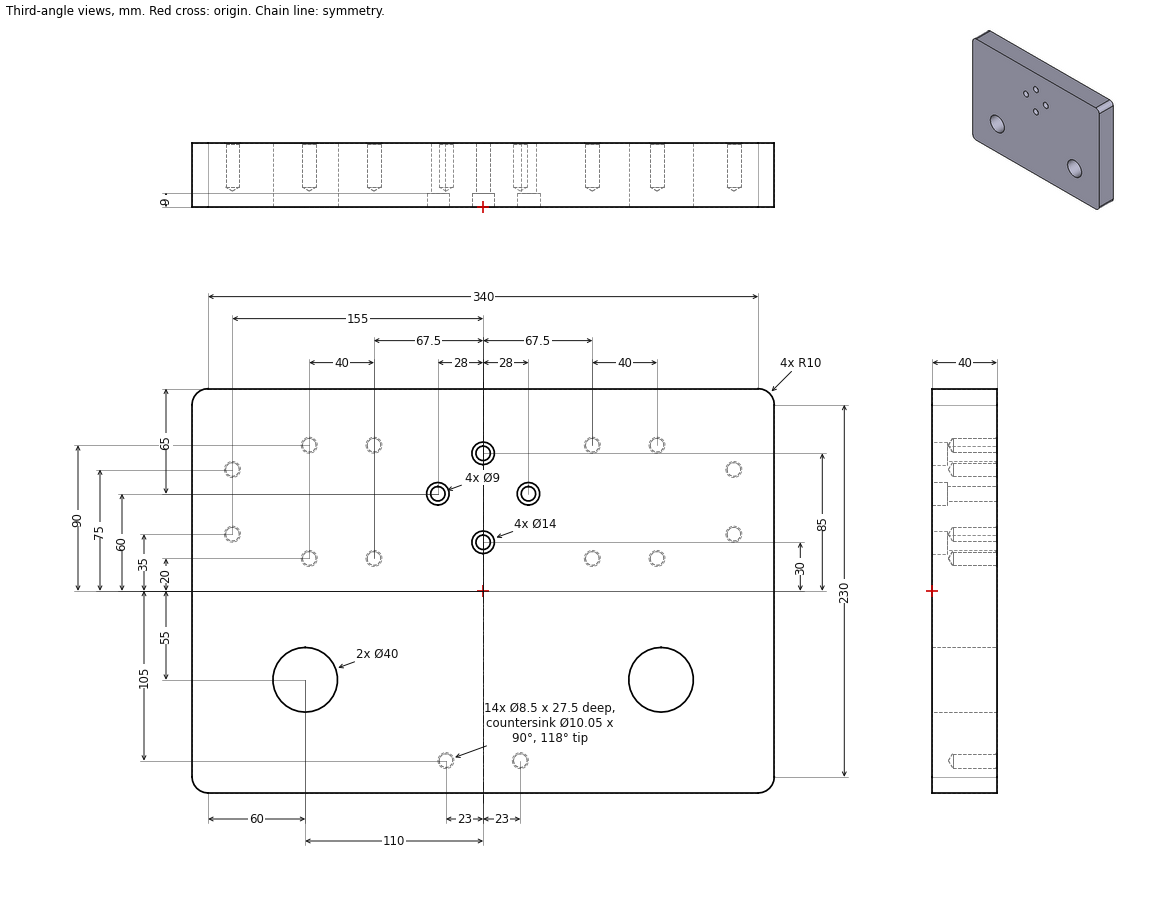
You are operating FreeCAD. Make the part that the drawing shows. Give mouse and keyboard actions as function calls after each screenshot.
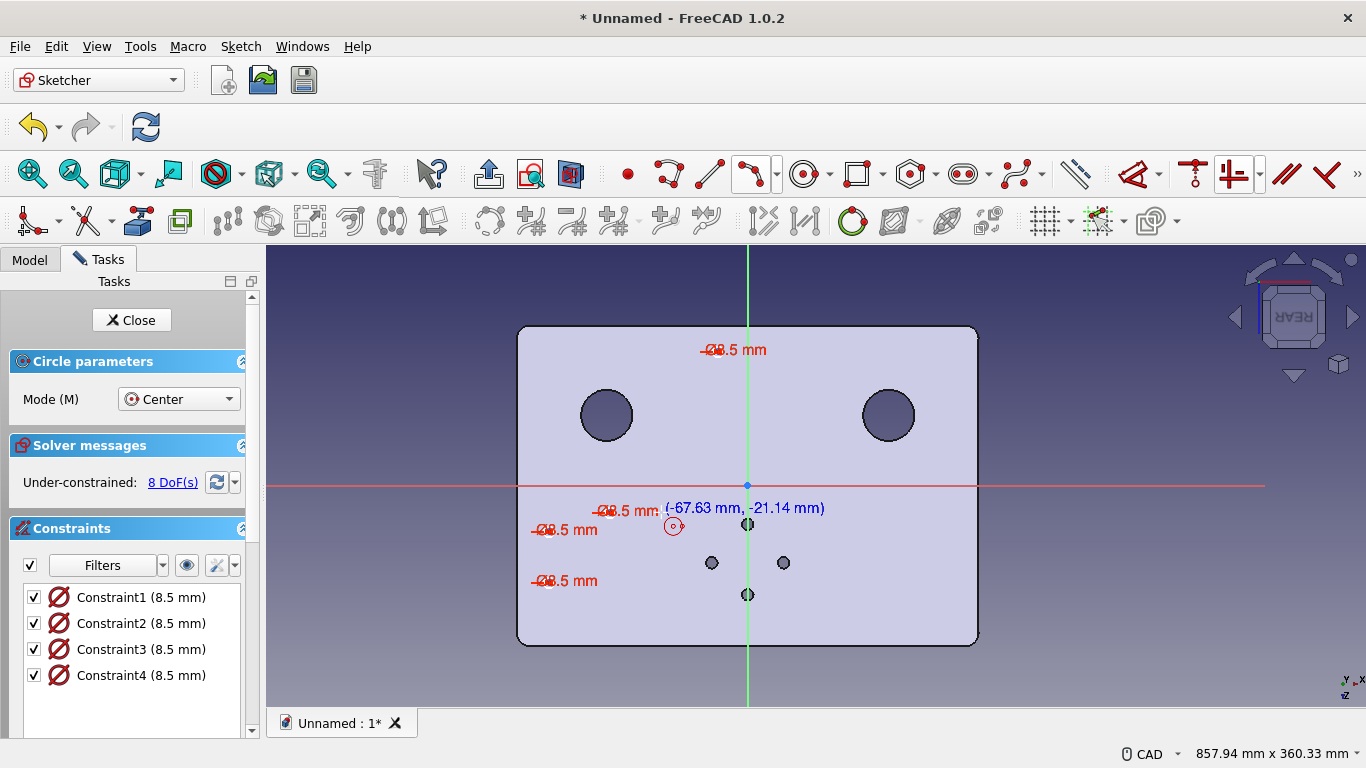
click(661, 512)
move(665, 508)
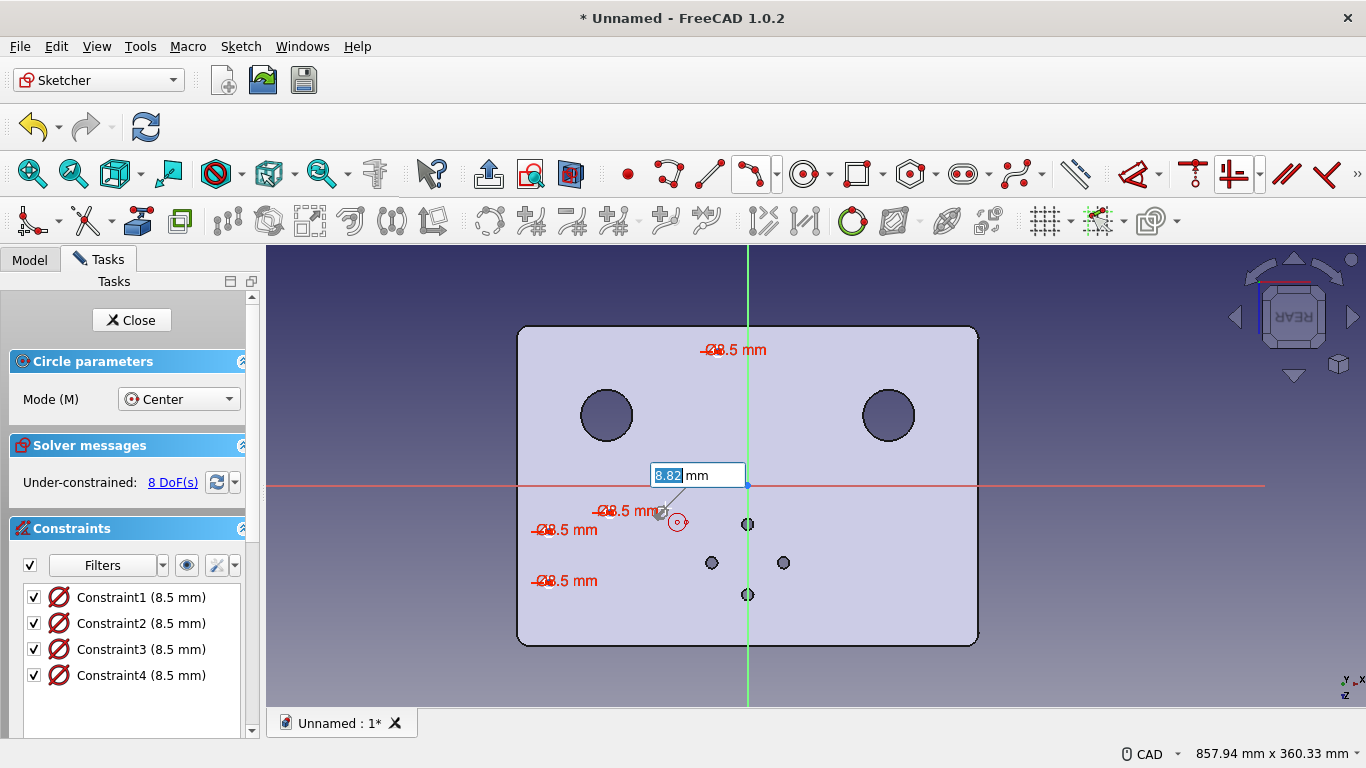
text(8.5)
key(Return)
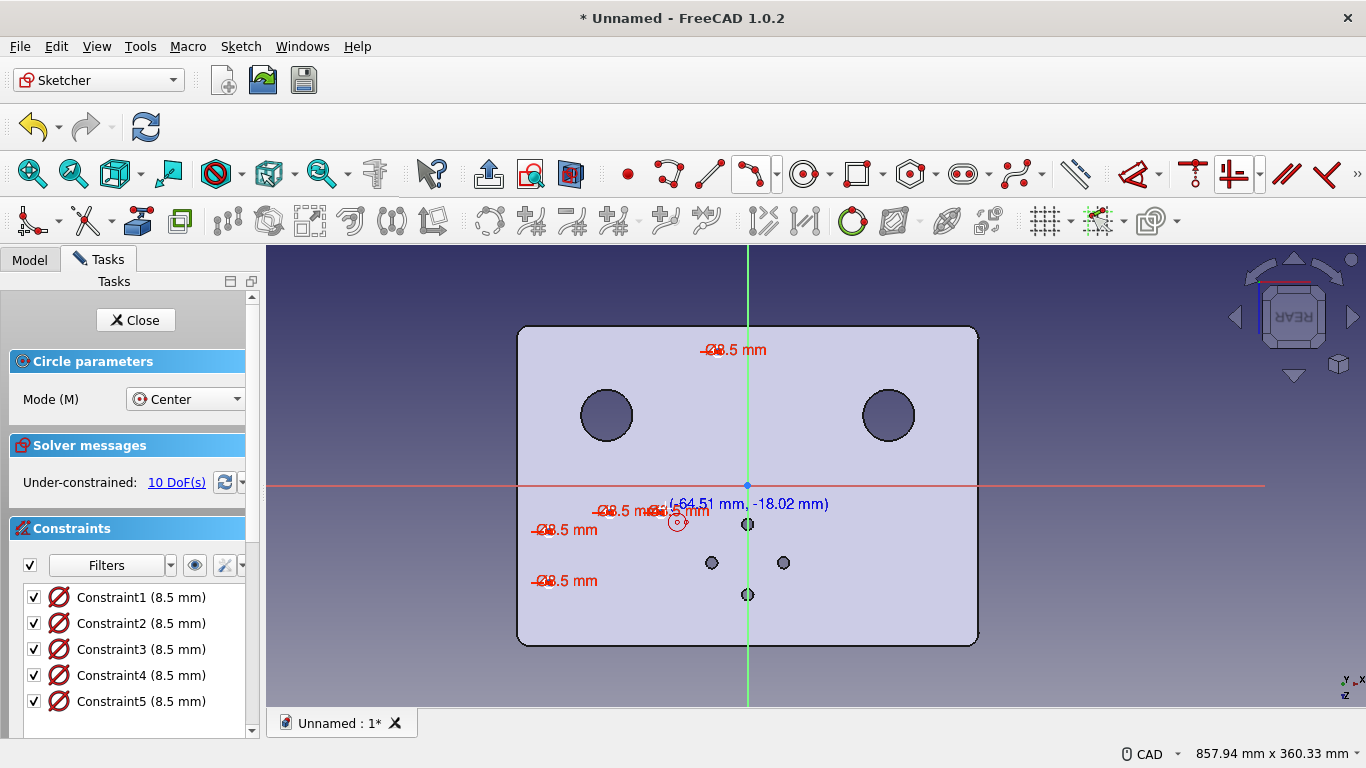
scroll(610, 601, up, 8)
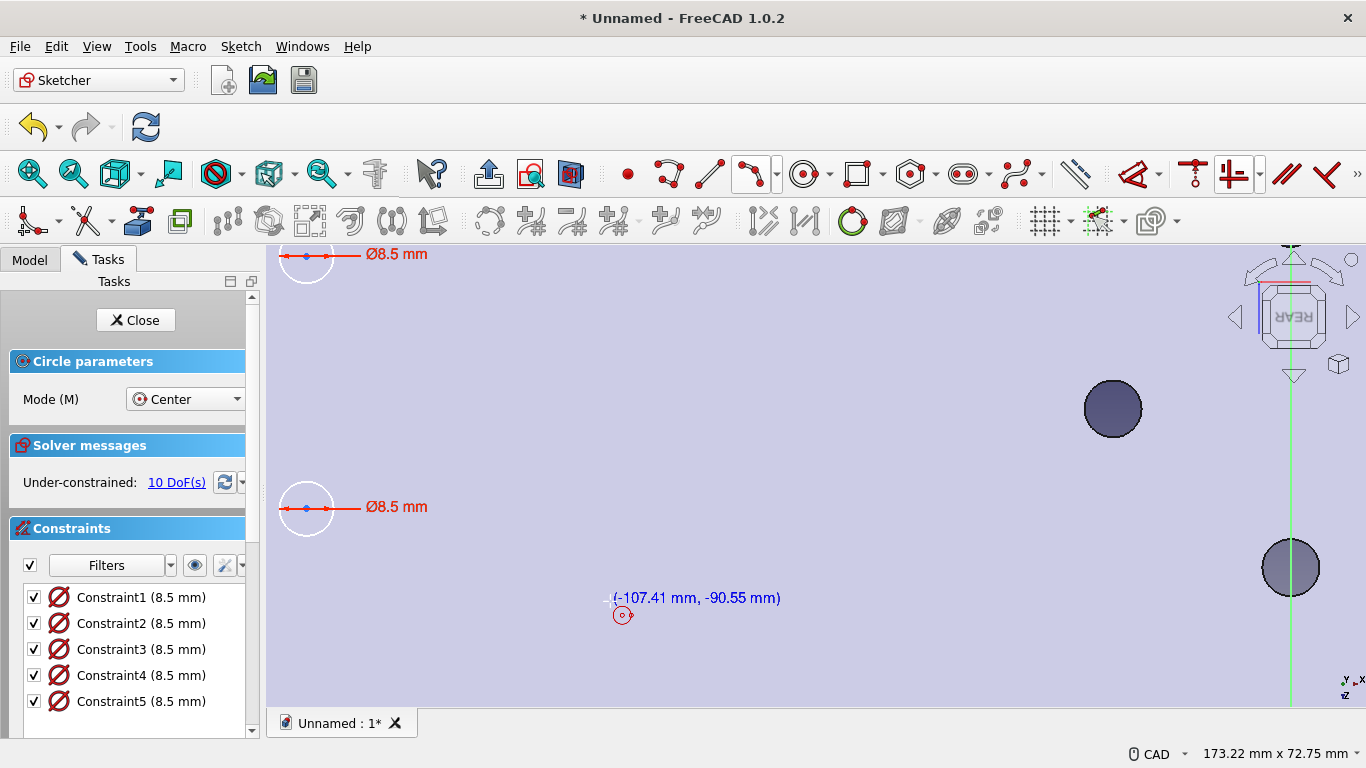
scroll(610, 601, down, 8)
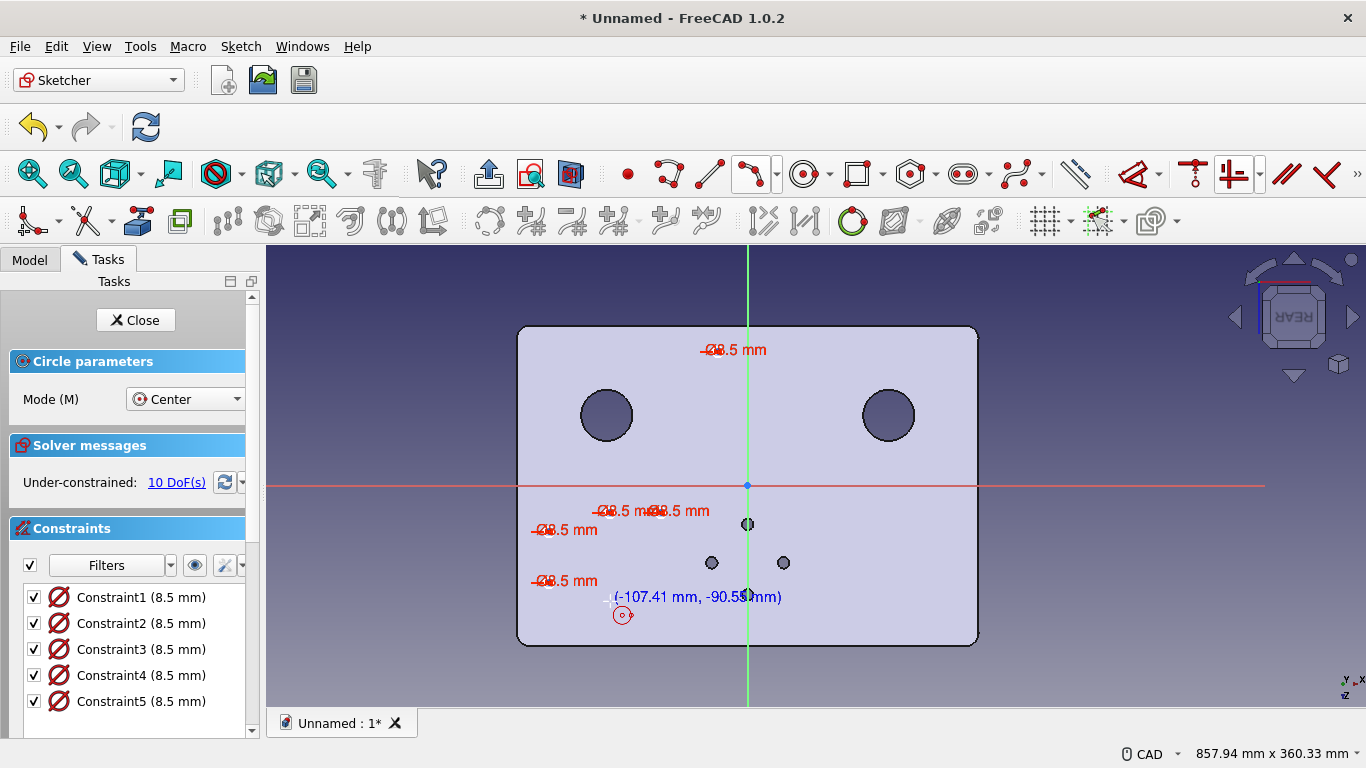
click(610, 601)
move(614, 597)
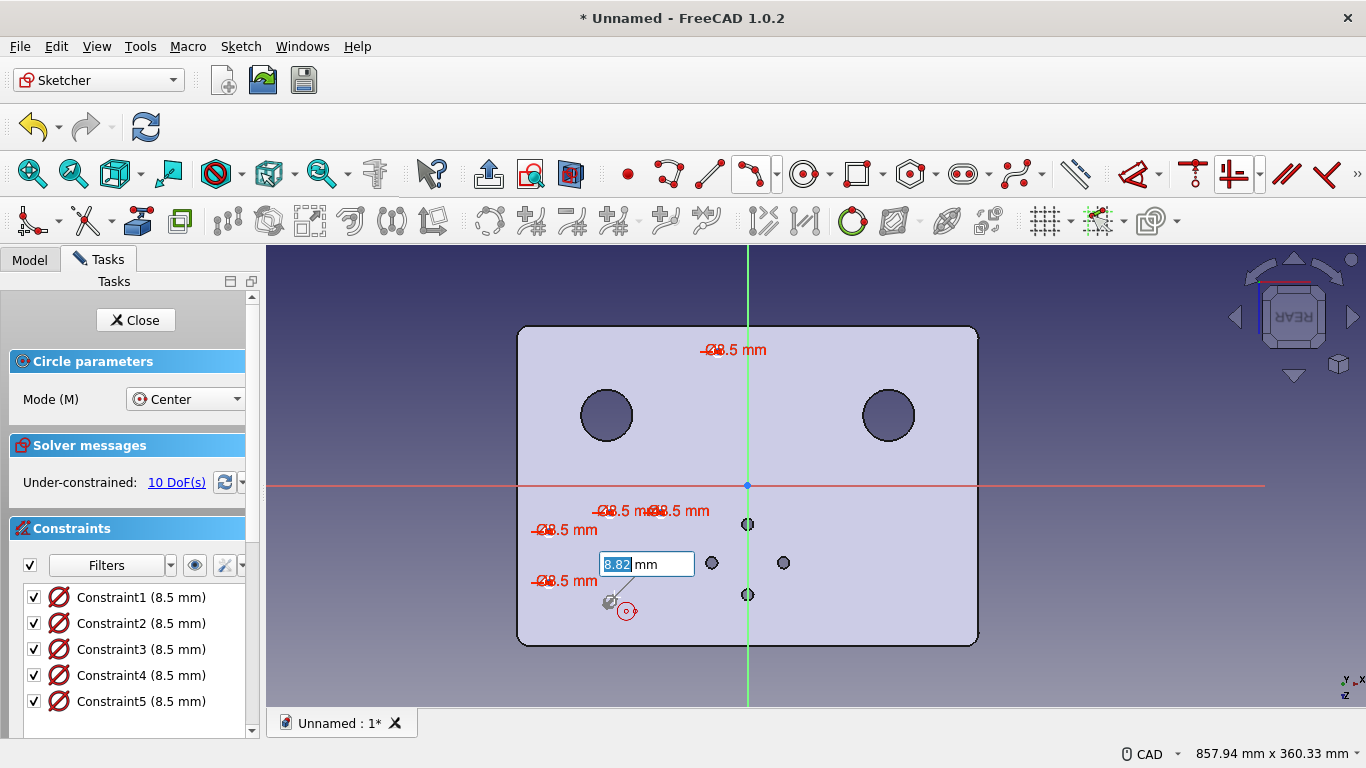
text(8.5)
key(Return)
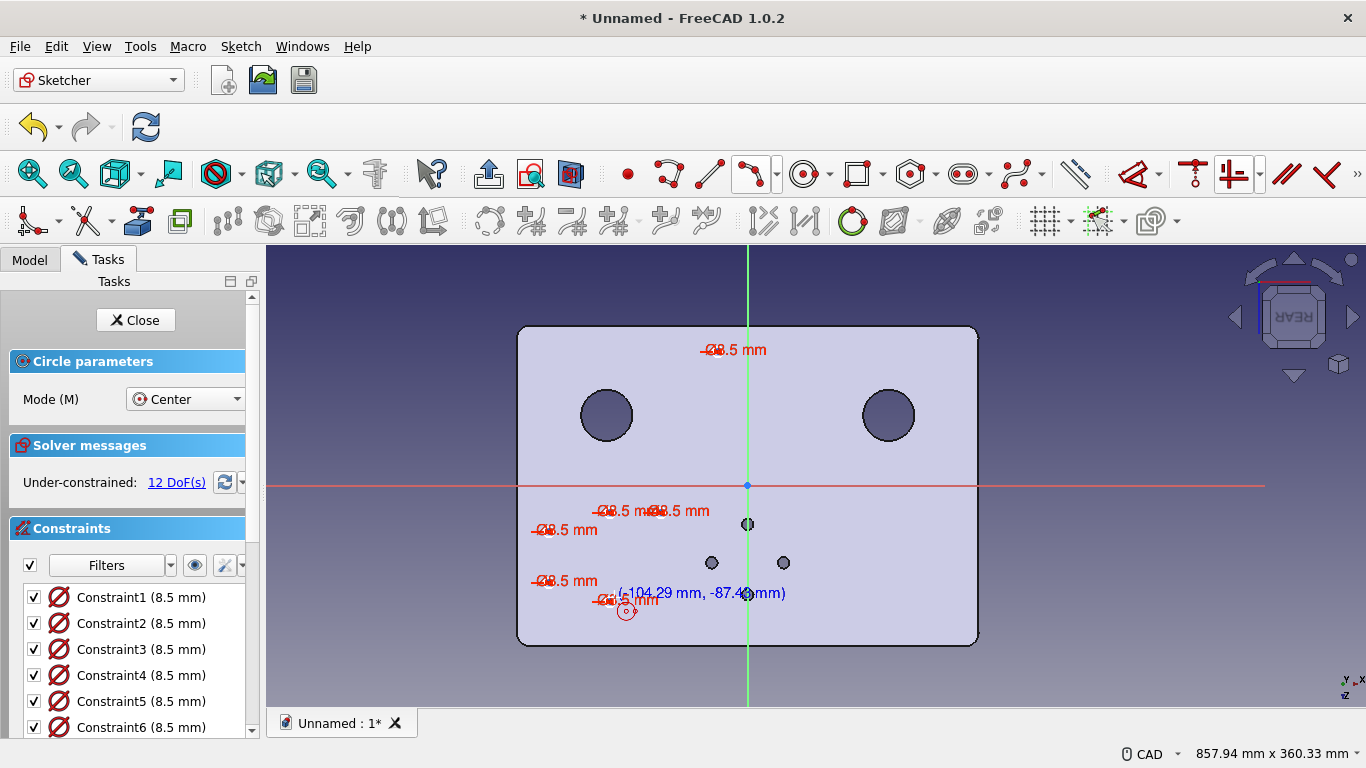
scroll(661, 601, up, 8)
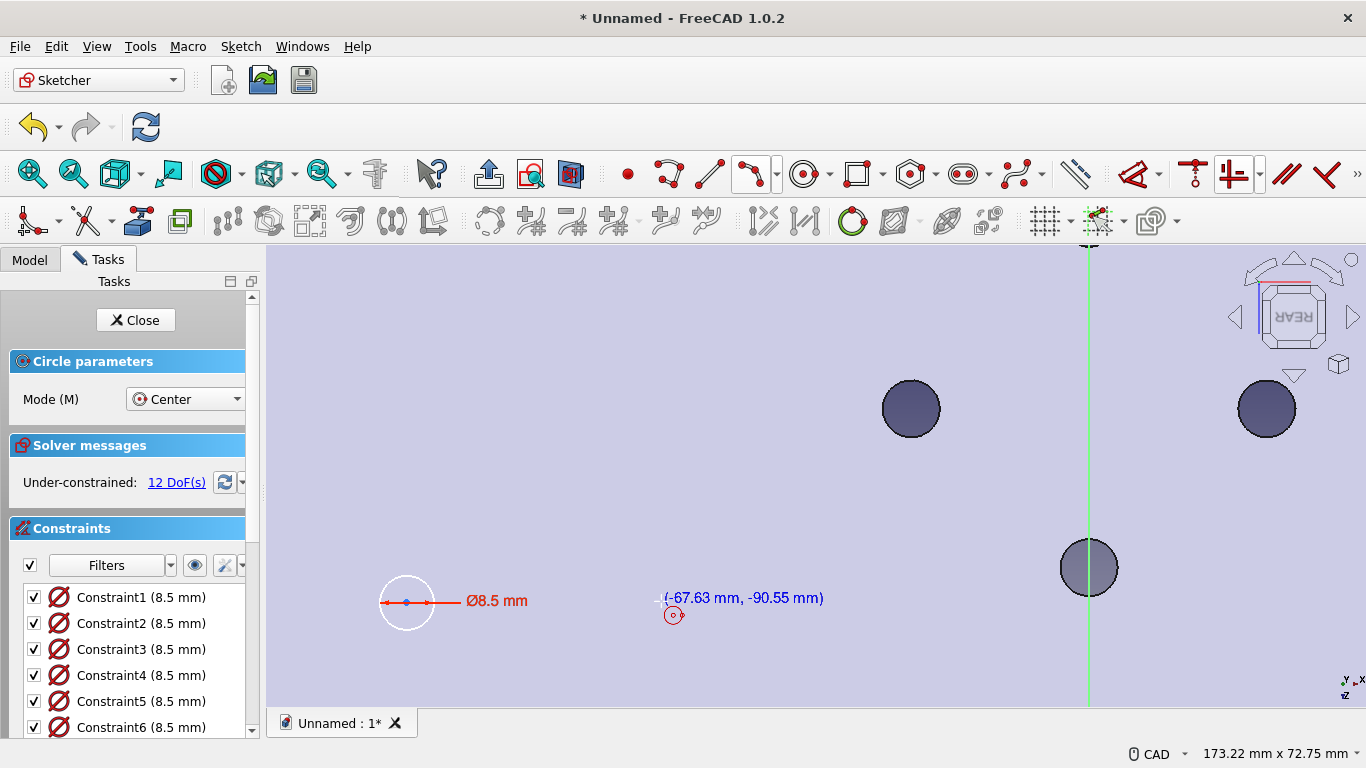
scroll(661, 601, down, 8)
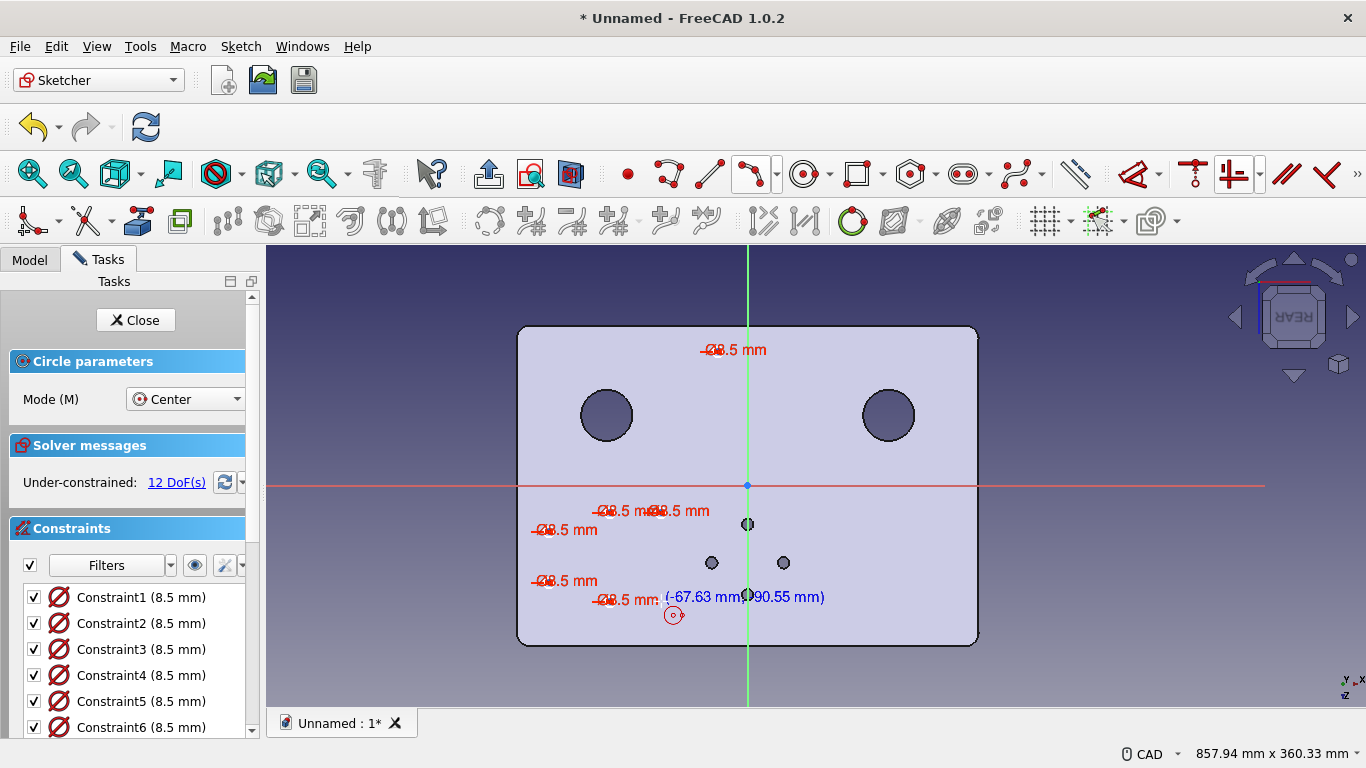
click(661, 601)
move(665, 597)